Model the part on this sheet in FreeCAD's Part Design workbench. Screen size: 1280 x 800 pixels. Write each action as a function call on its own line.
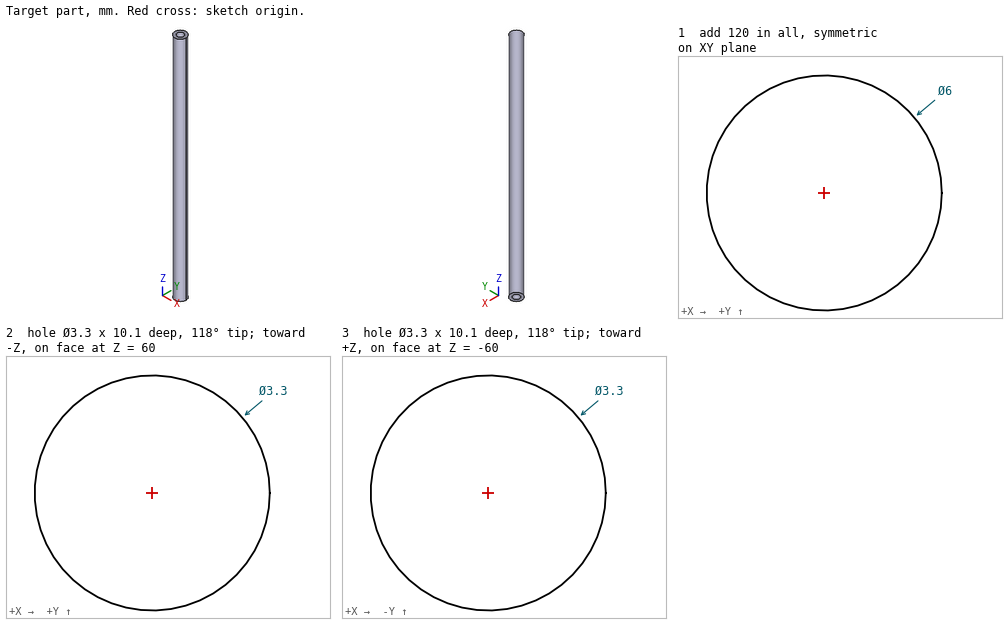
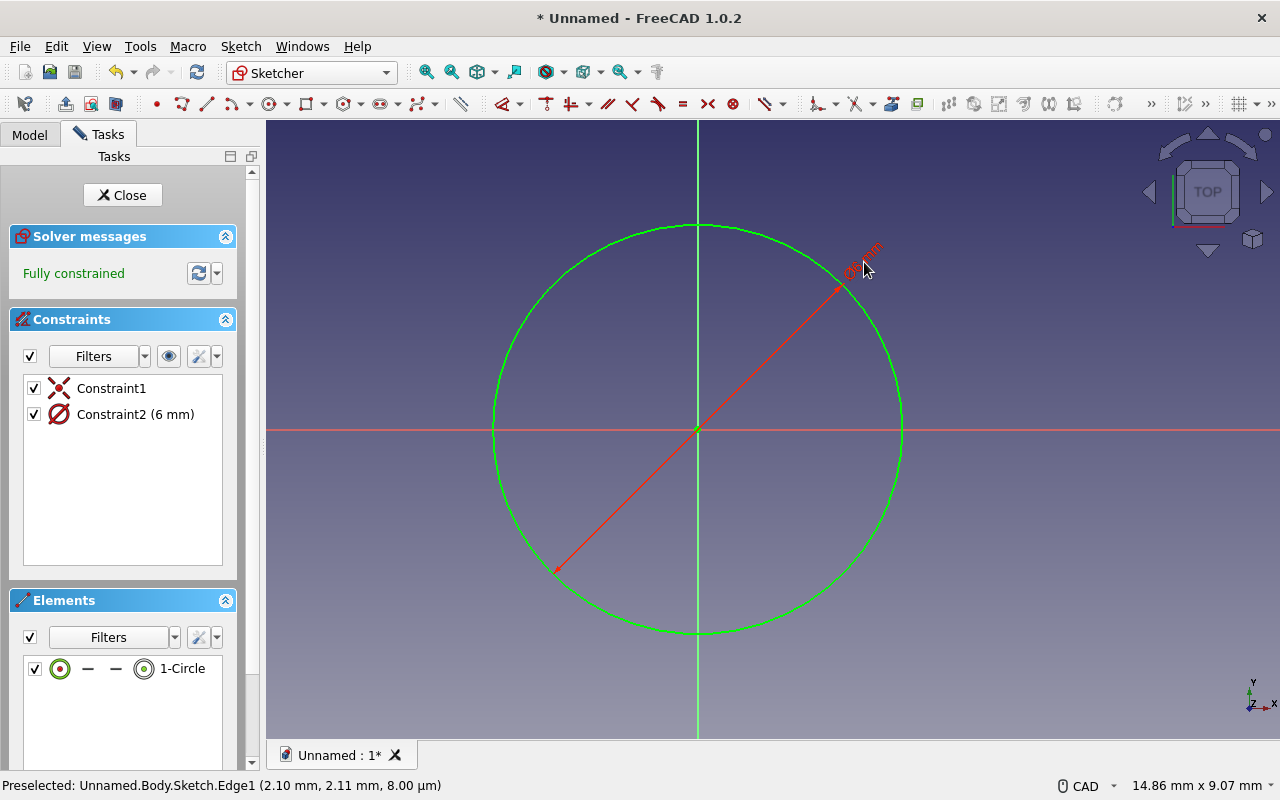
click(123, 195)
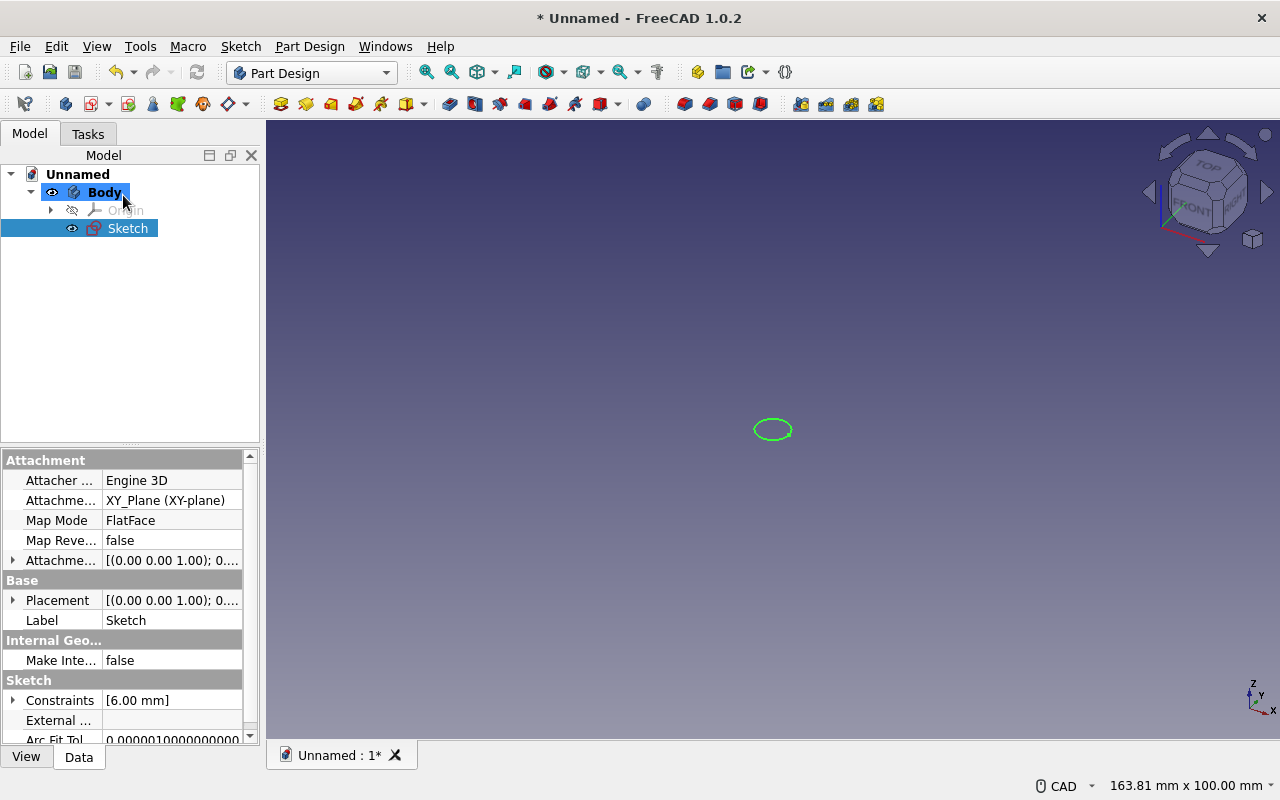
click(281, 104)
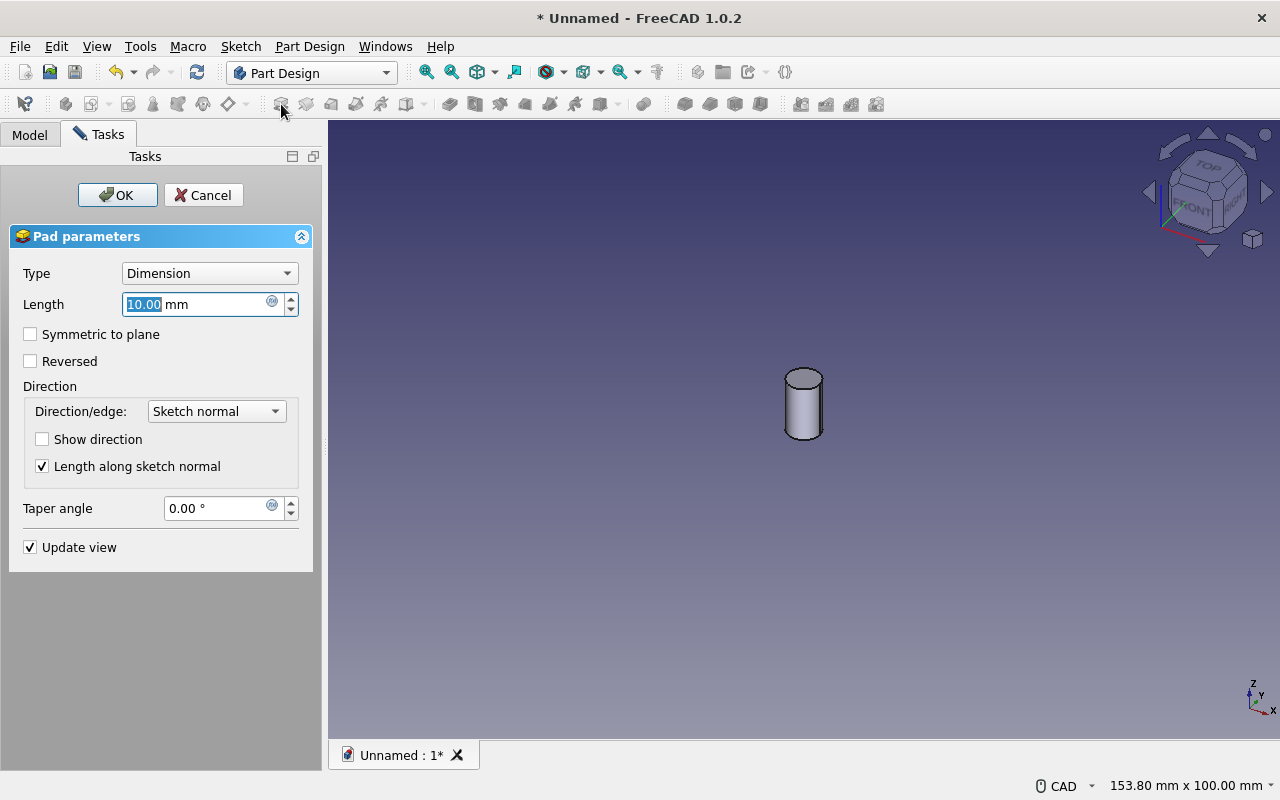
text(120)
key(Tab)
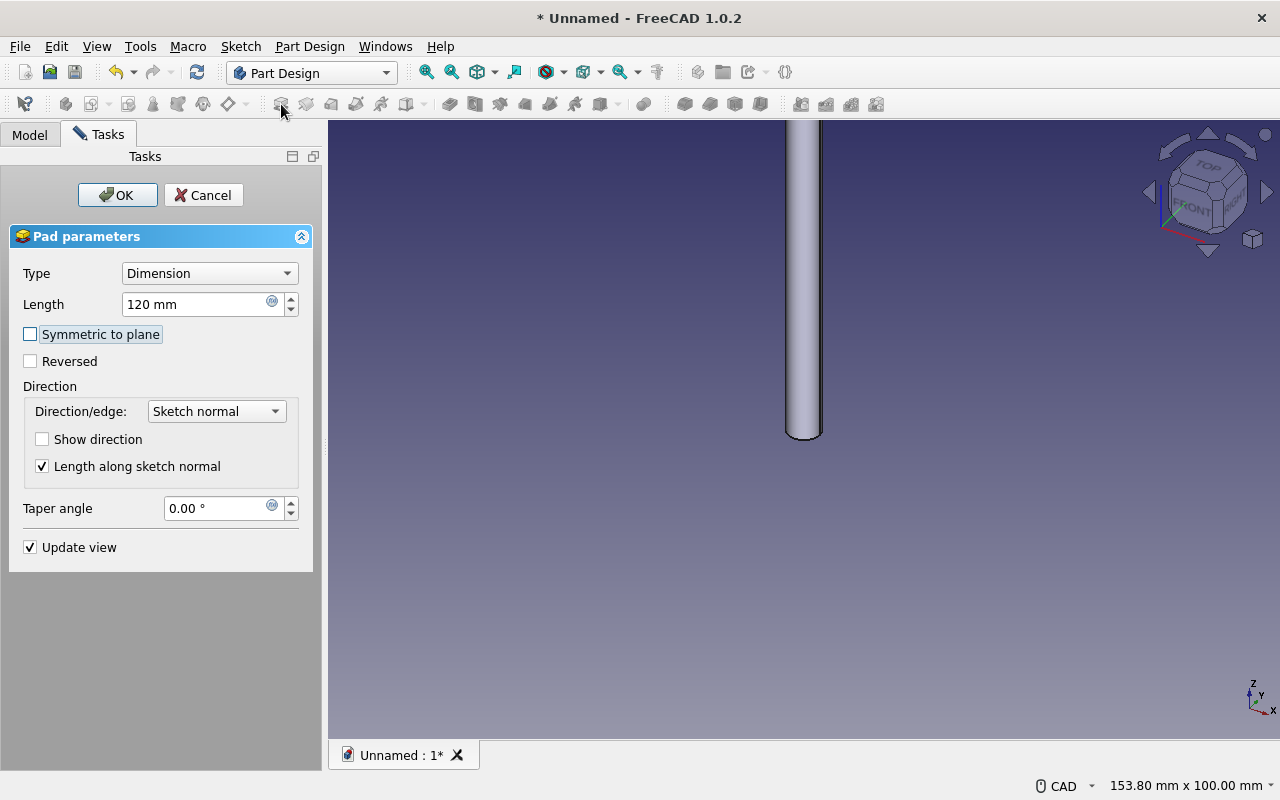
click(31, 334)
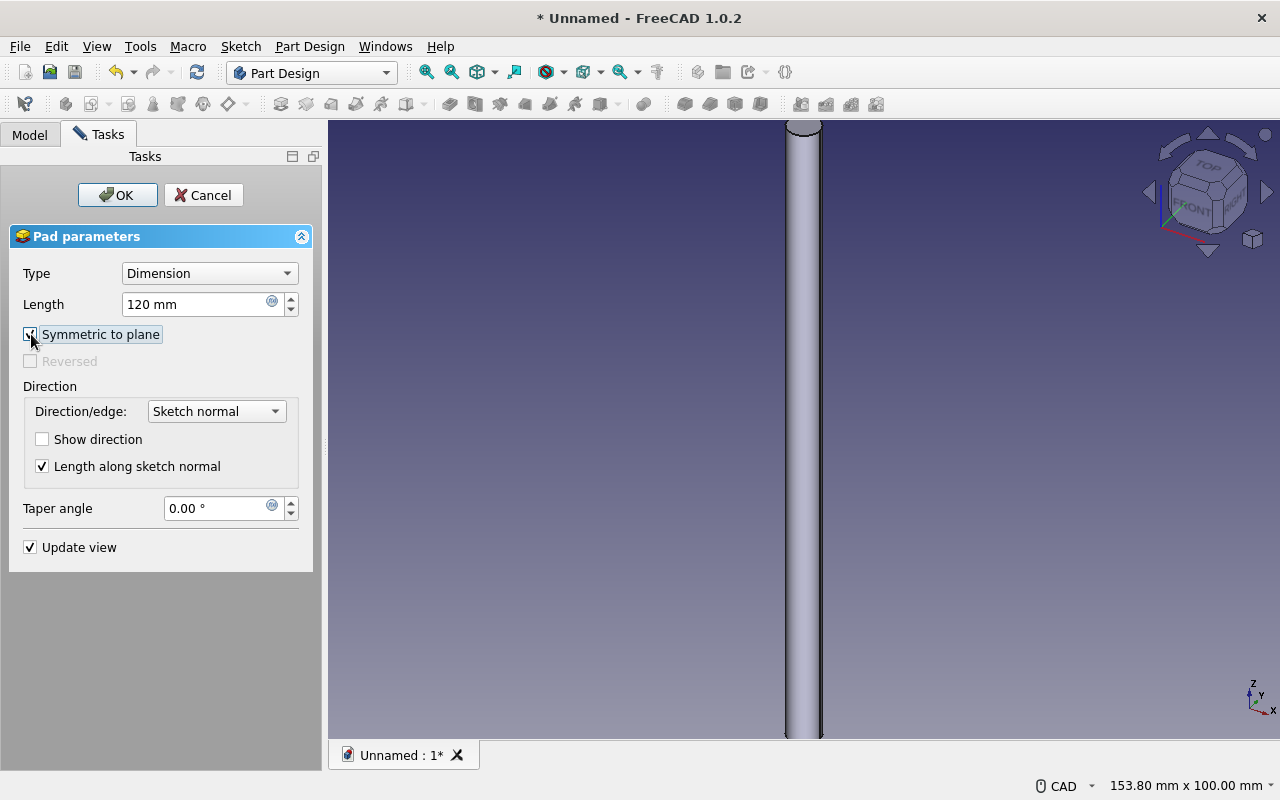
click(118, 195)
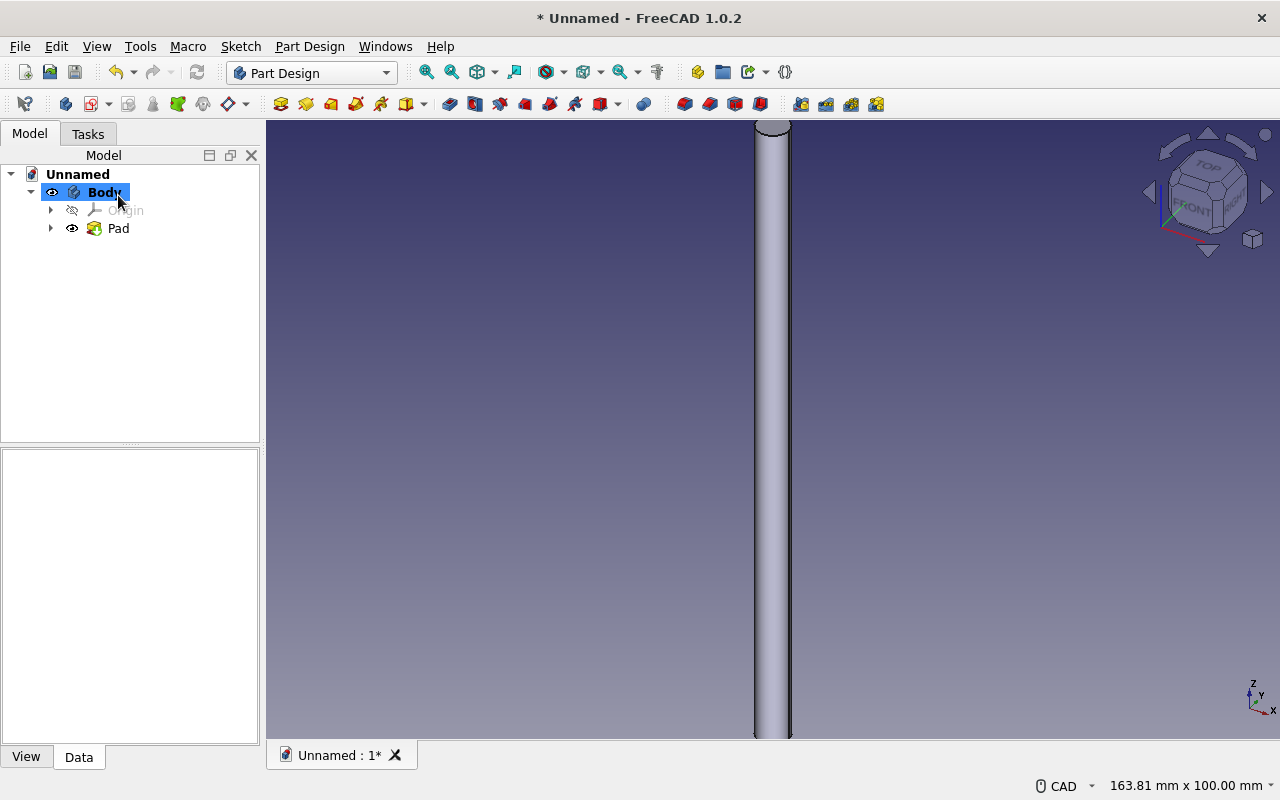
key(v)
key(f)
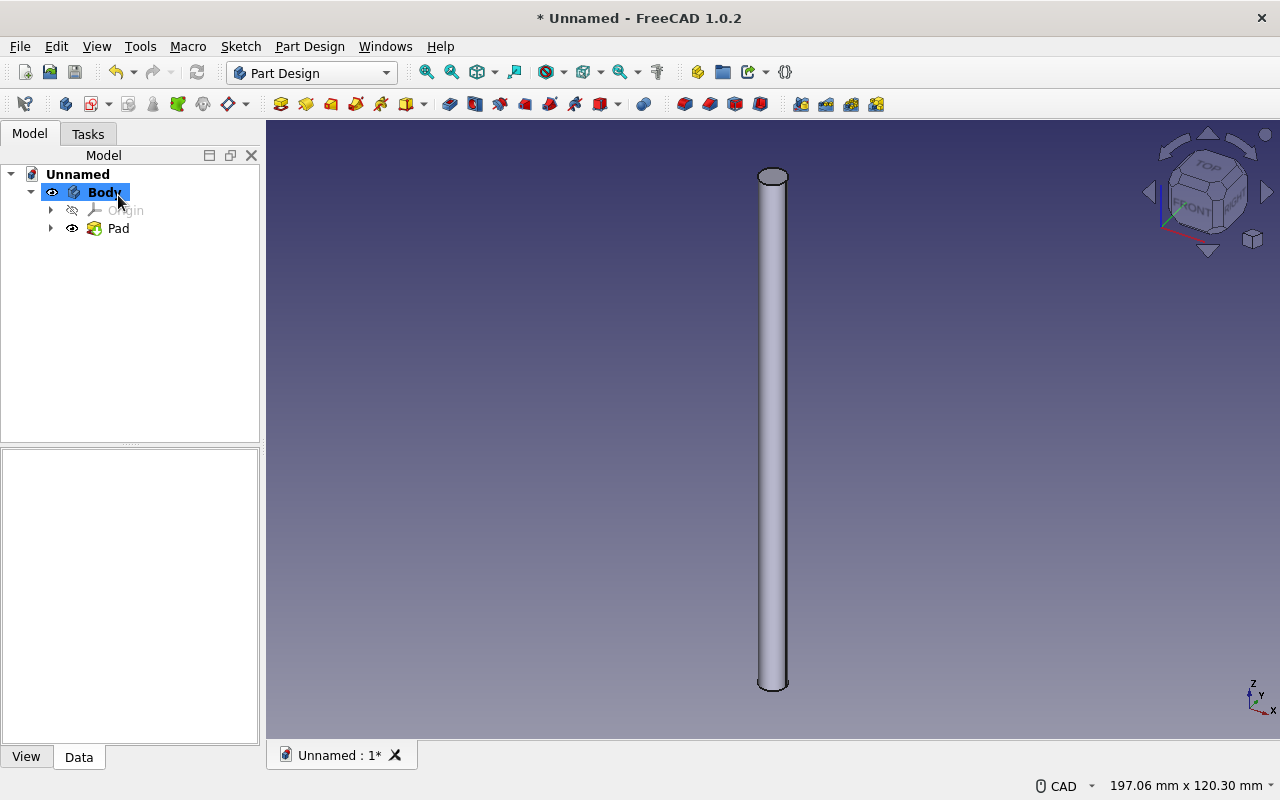
click(773, 176)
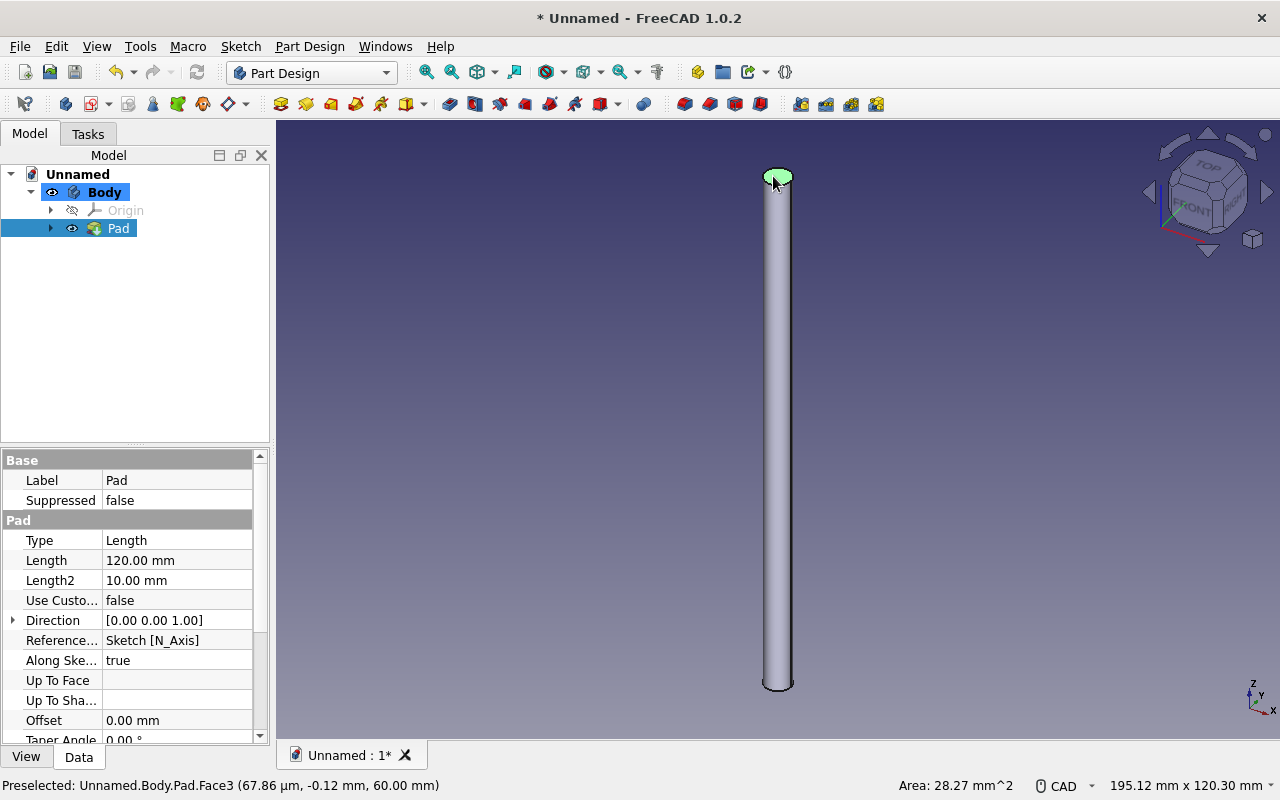
click(90, 104)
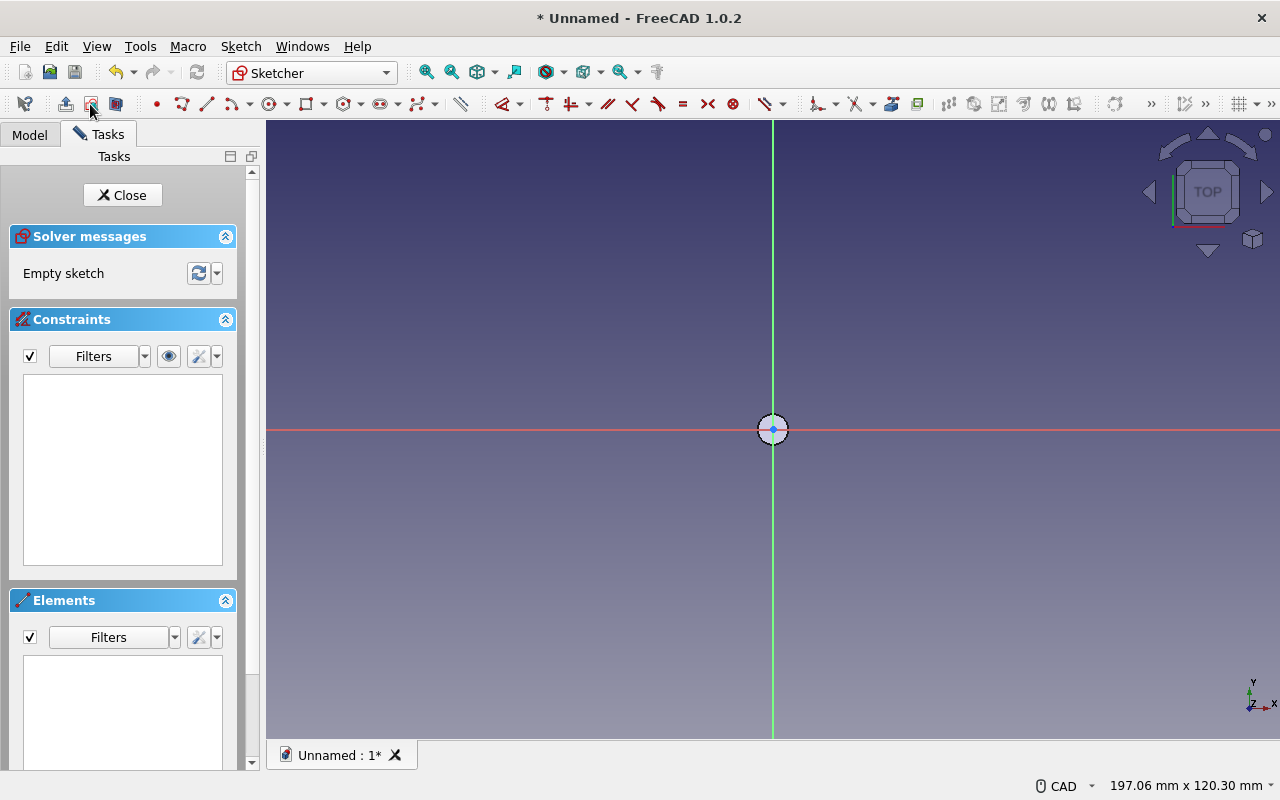
scroll(777, 430, up, 15)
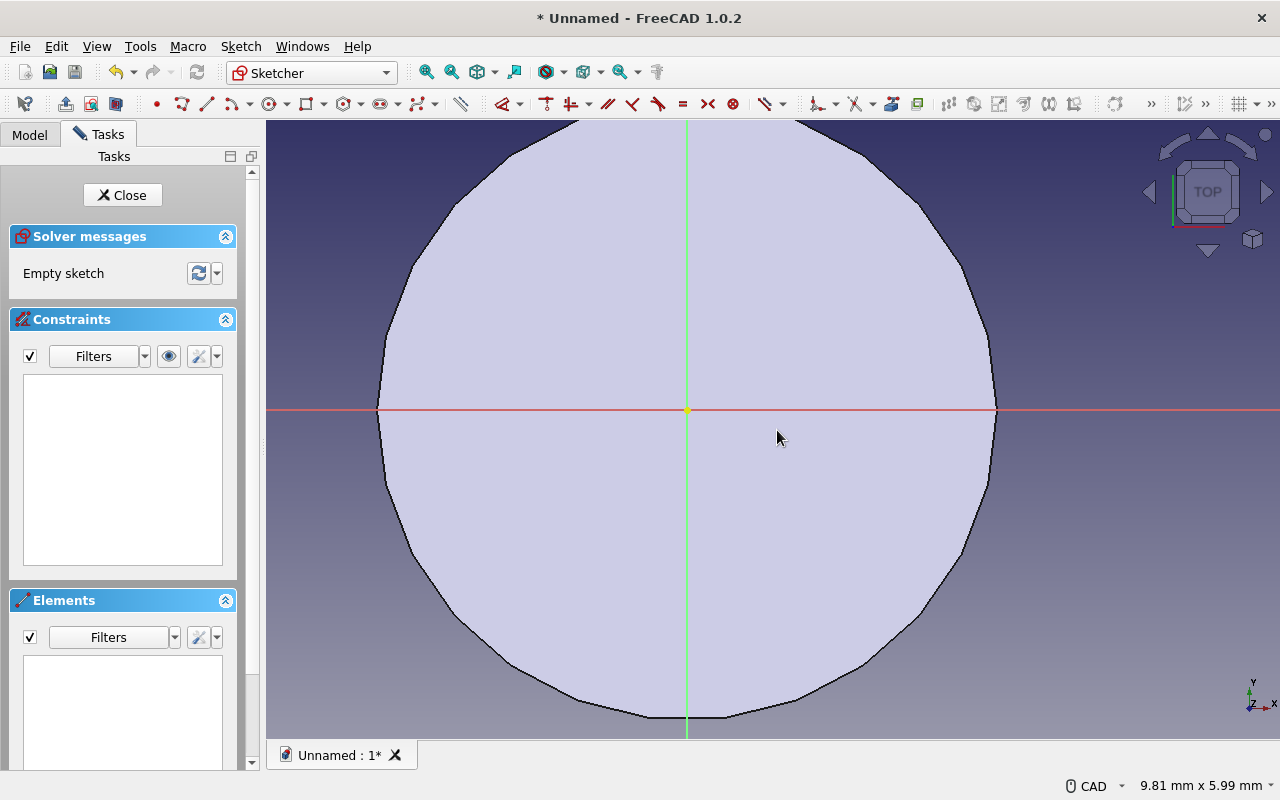
click(268, 104)